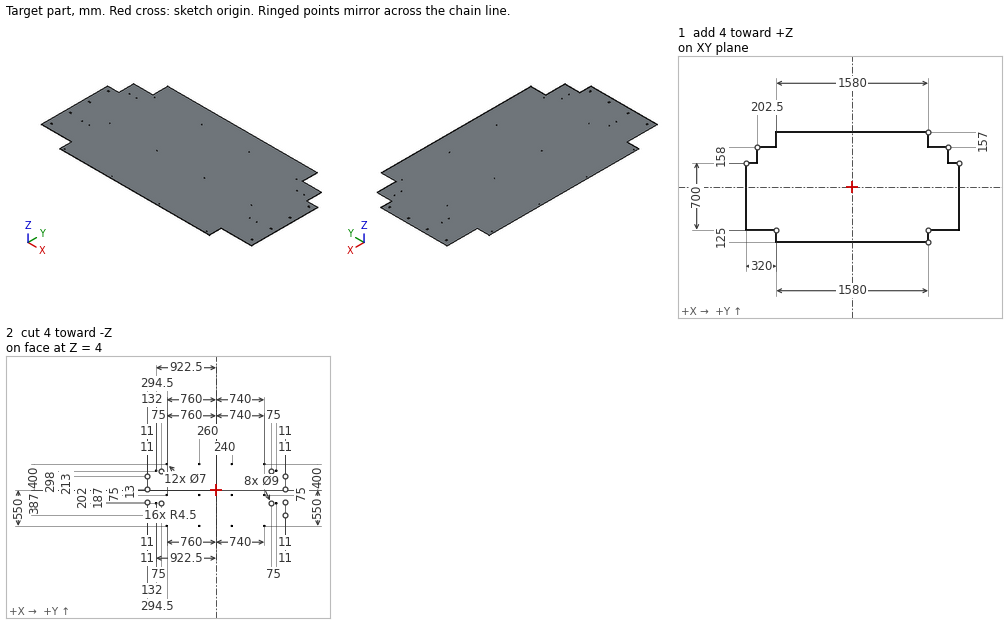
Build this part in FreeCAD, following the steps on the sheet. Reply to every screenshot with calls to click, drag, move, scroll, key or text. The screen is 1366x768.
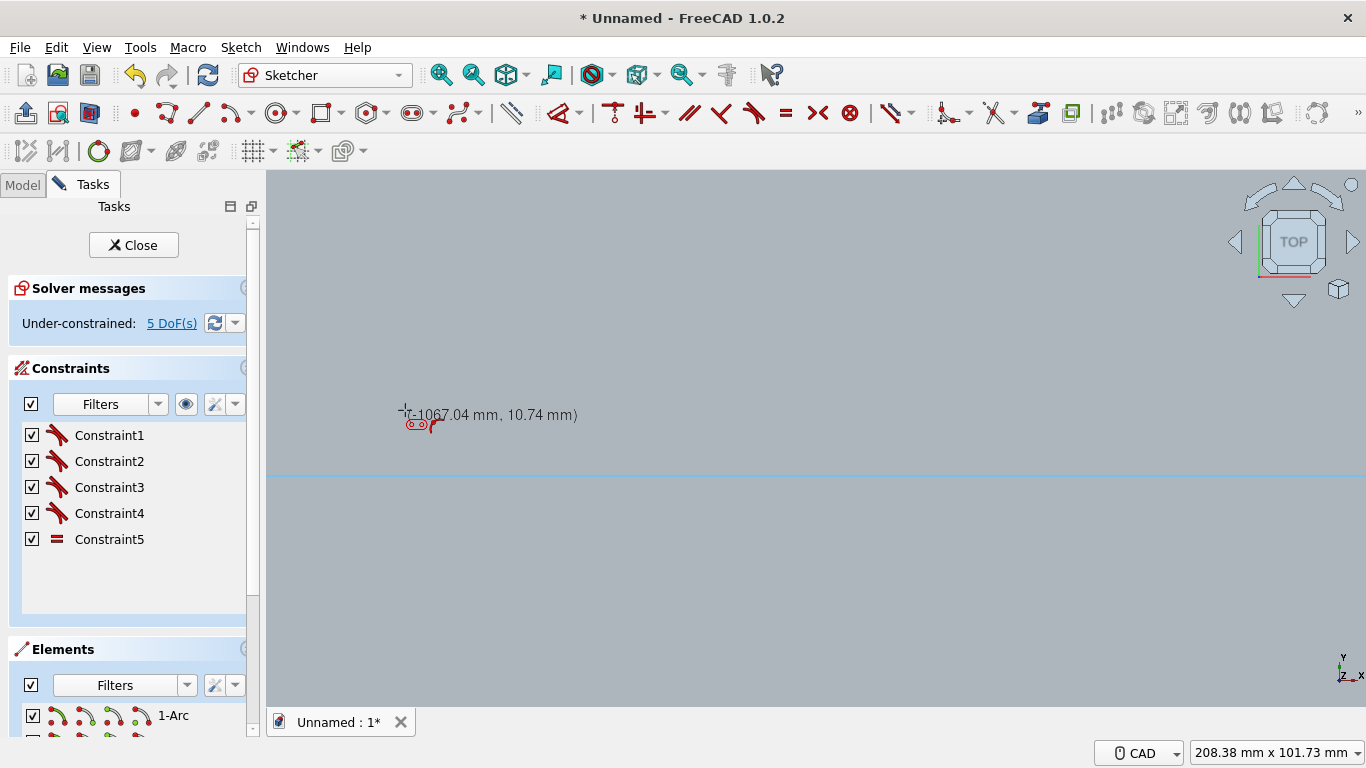
scroll(405, 410, down, 14)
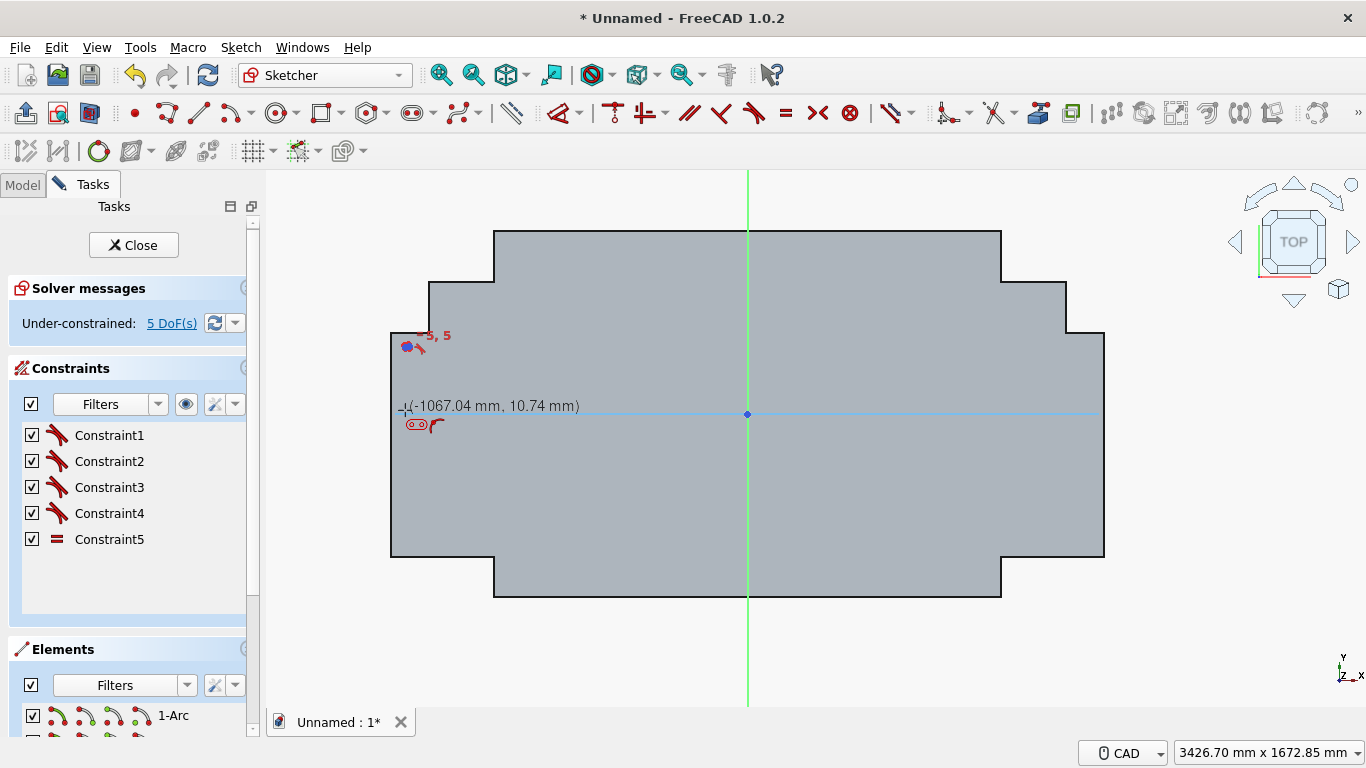
scroll(405, 410, up, 7)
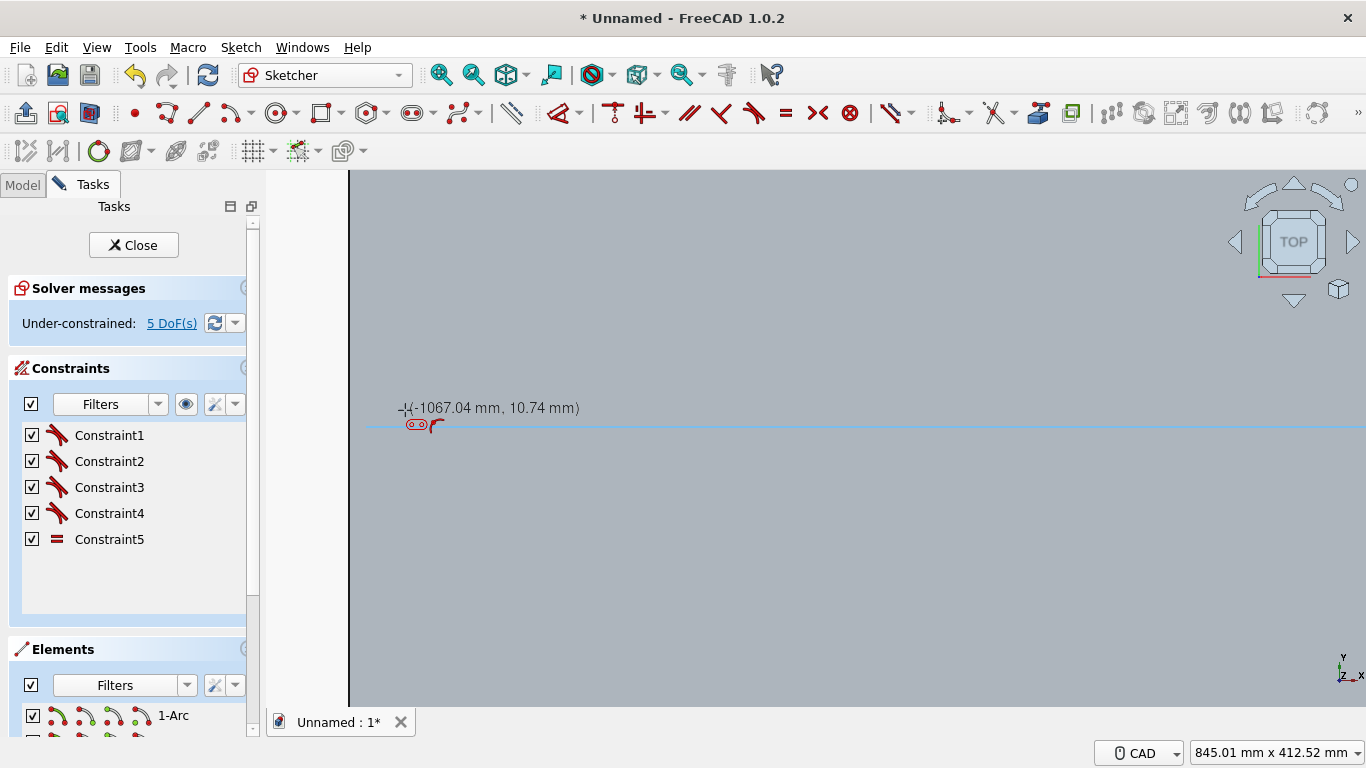
click(407, 410)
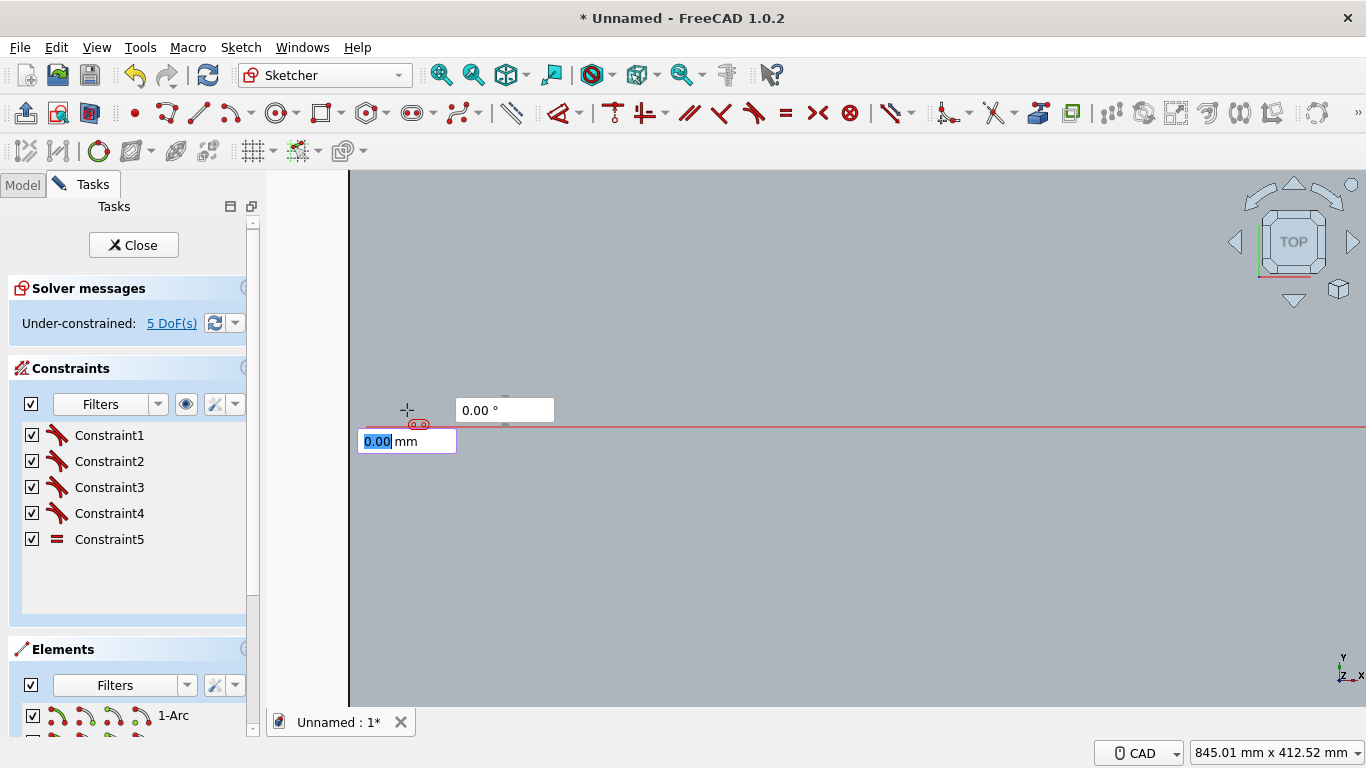
click(421, 410)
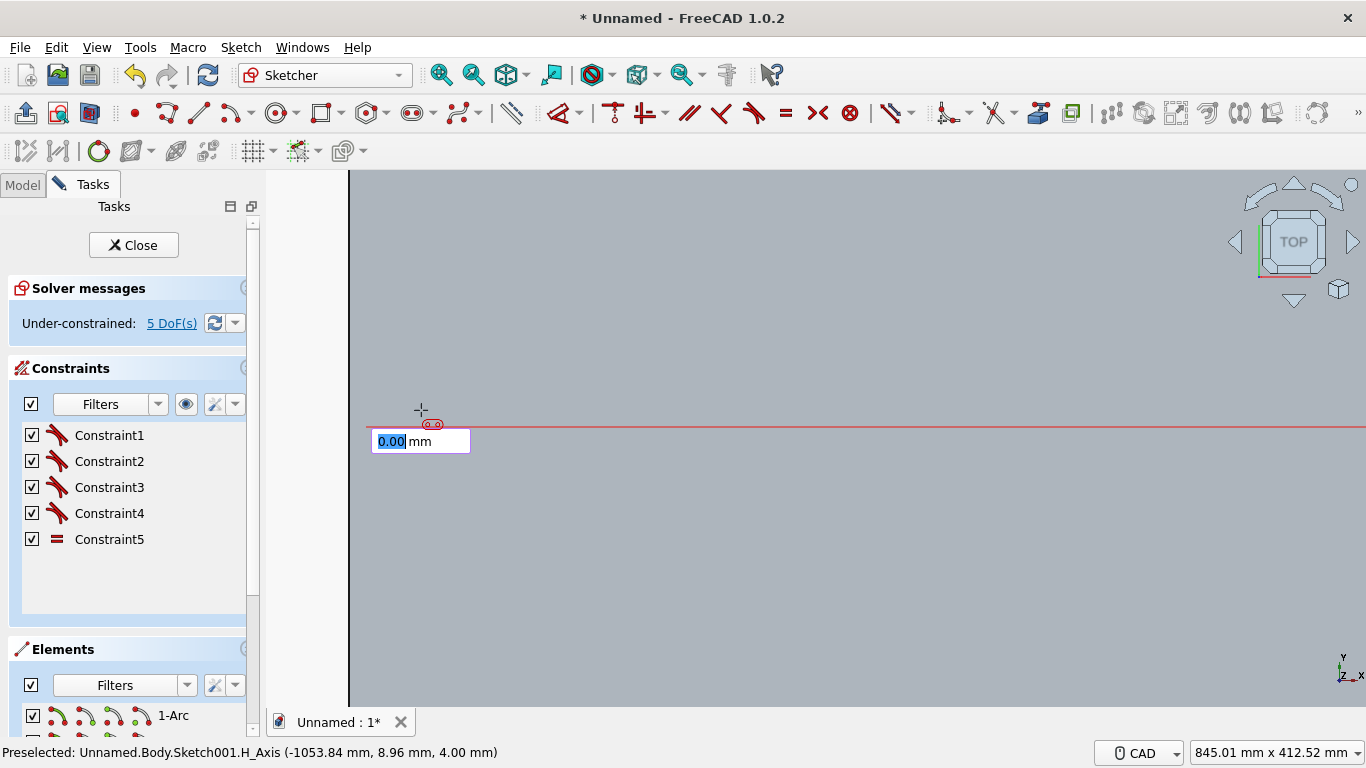
scroll(414, 404, up, 5)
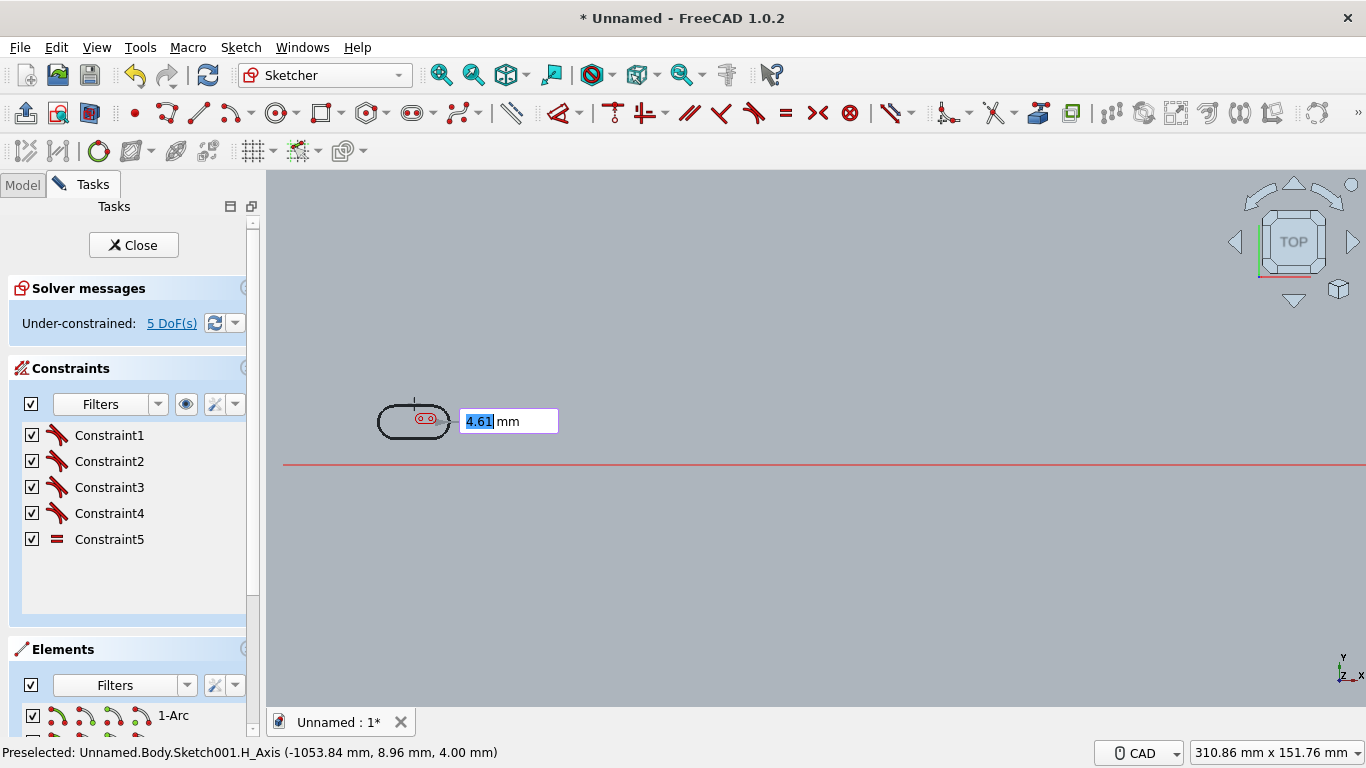
click(413, 403)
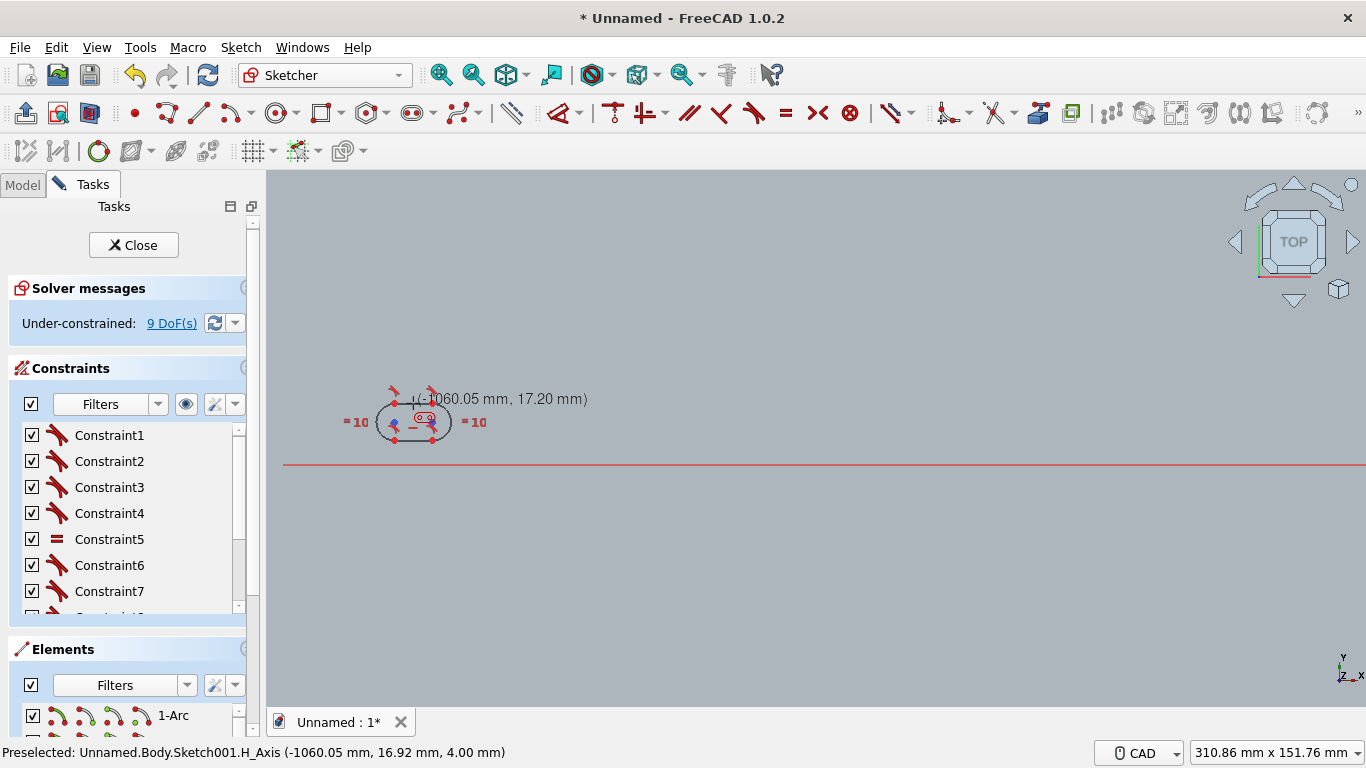
scroll(407, 409, down, 12)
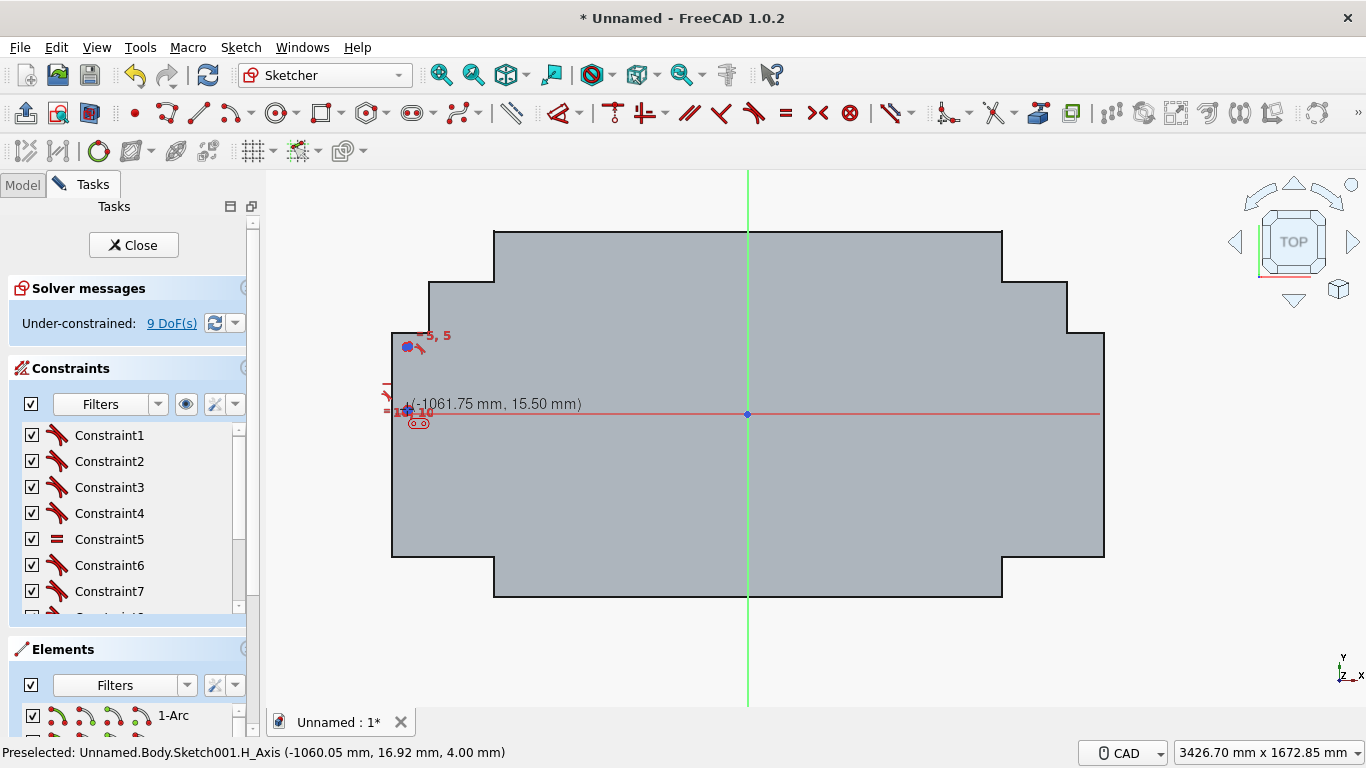
scroll(406, 475, up, 14)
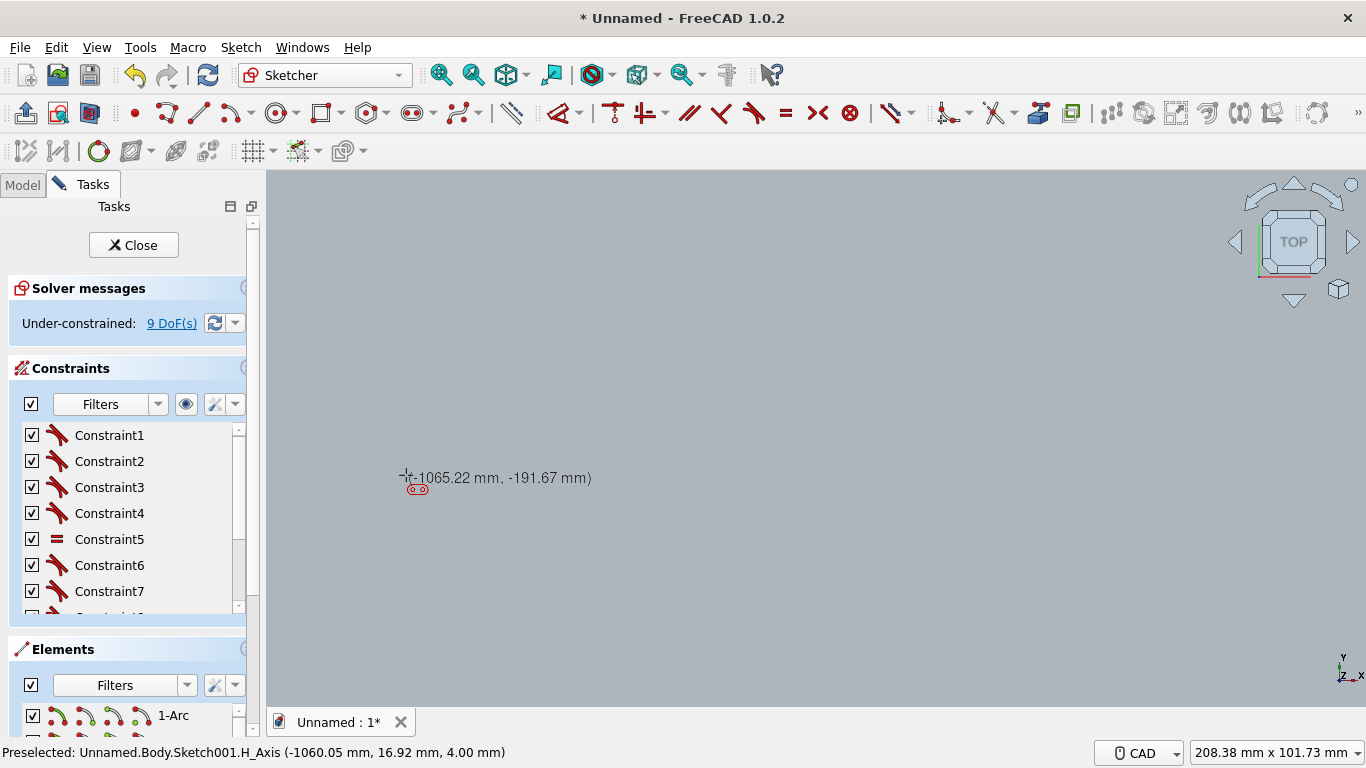
scroll(406, 476, down, 14)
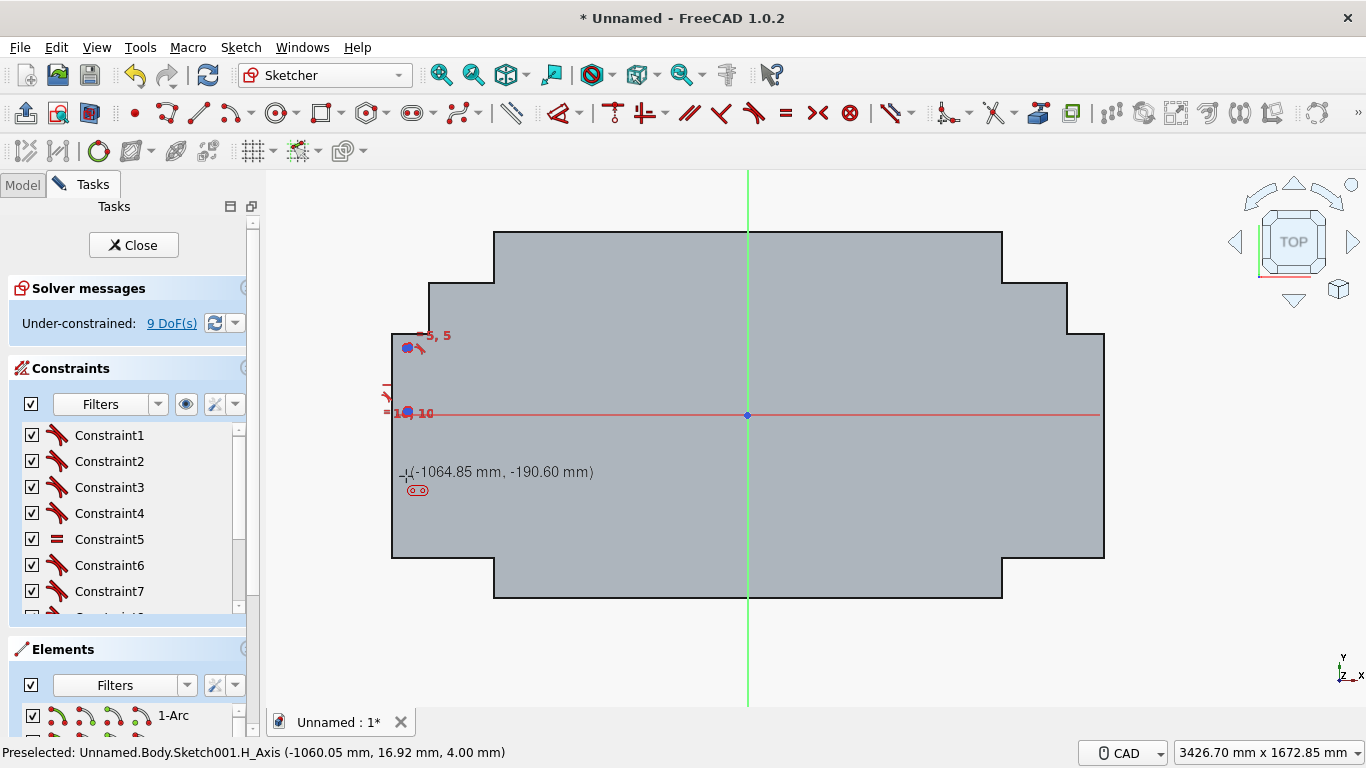
click(406, 475)